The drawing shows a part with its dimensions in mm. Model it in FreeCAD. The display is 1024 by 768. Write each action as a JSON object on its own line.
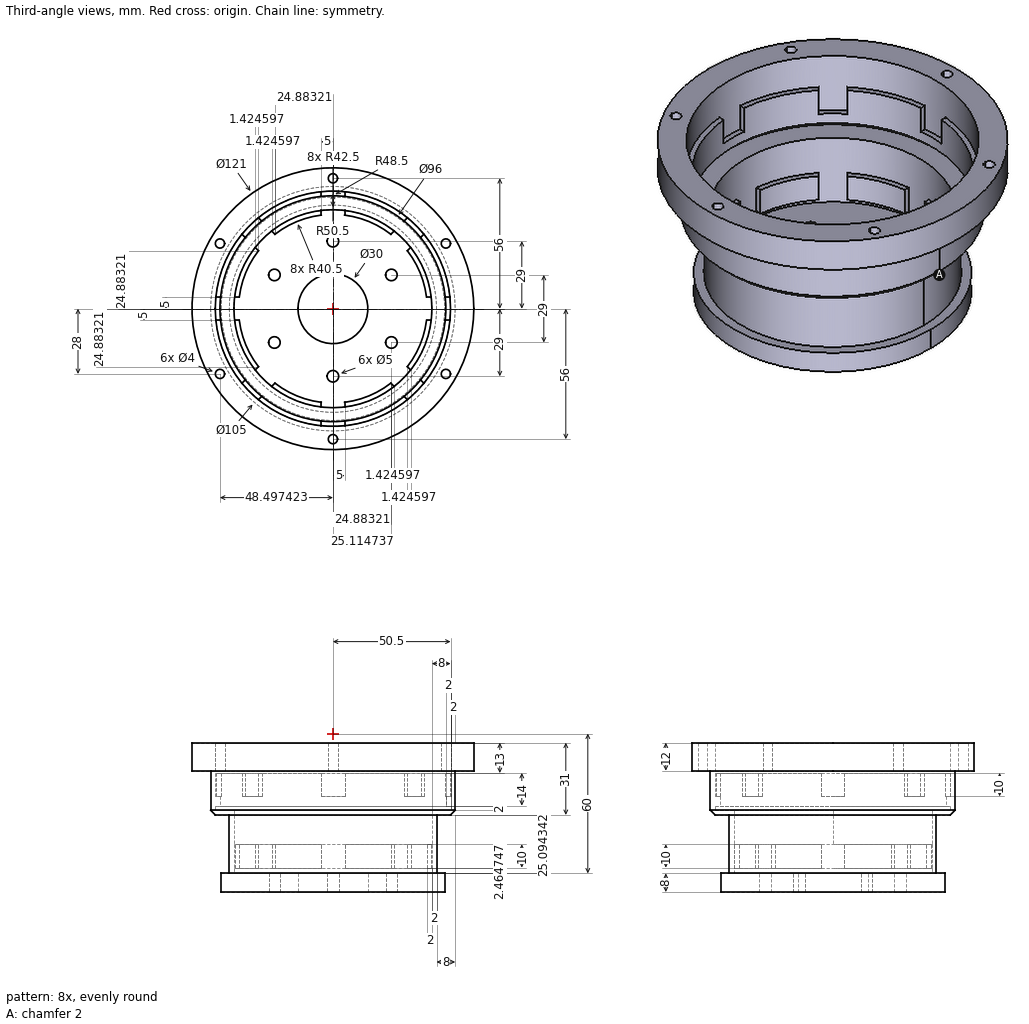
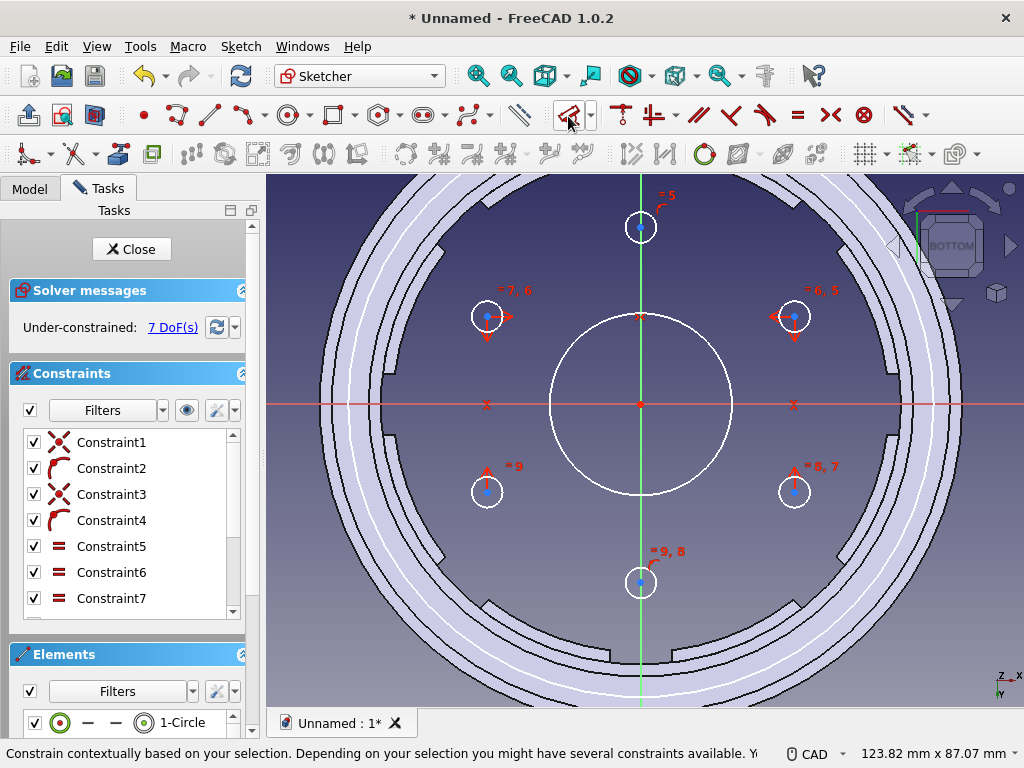
{"action": "left_click", "coordinate": [435, 612]}
{"action": "left_click", "coordinate": [412, 635]}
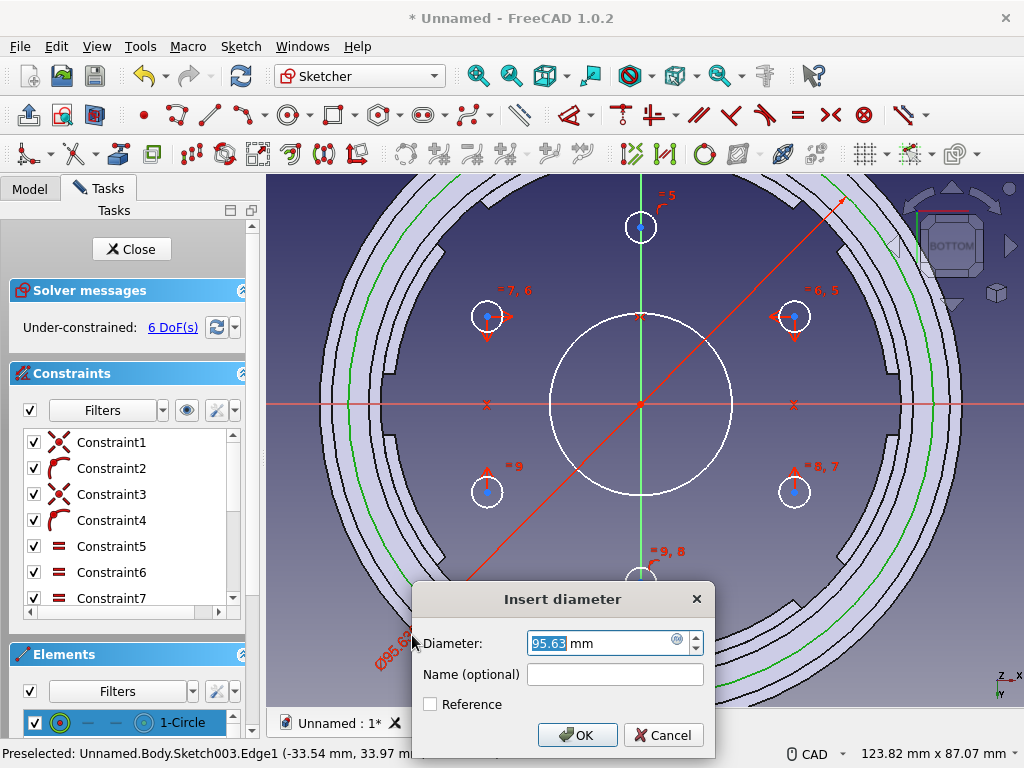
{"action": "type", "text": "96"}
{"action": "key", "text": "Return"}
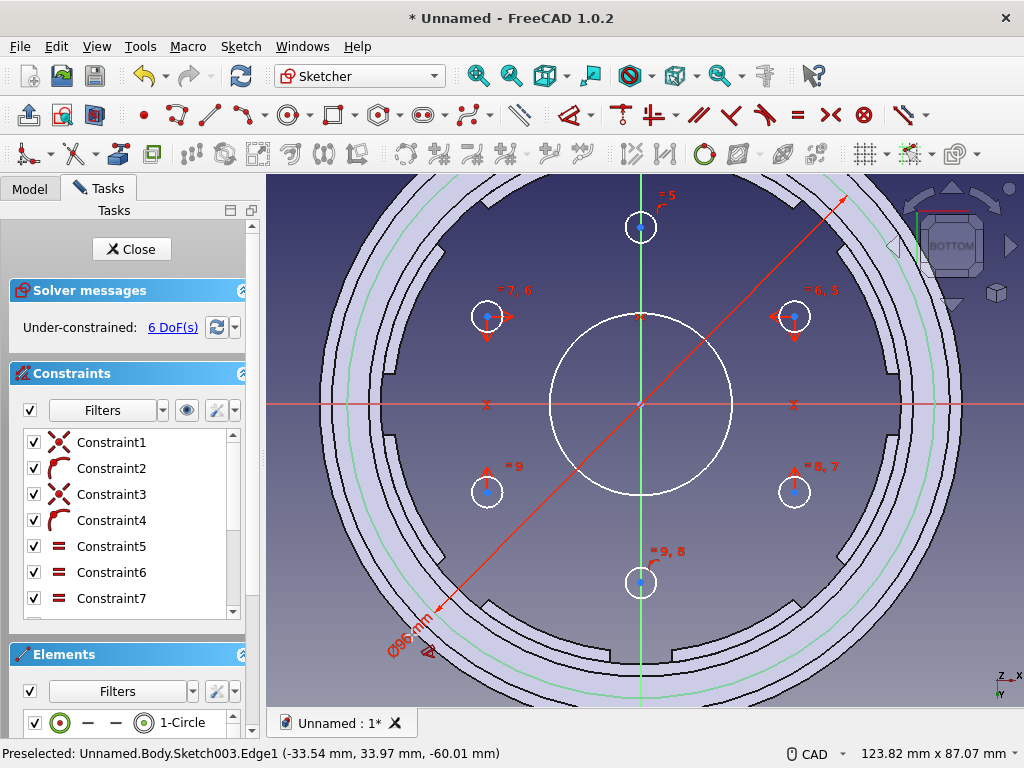
{"action": "scroll", "coordinate": [652, 217], "scroll_direction": "up", "scroll_amount": 2}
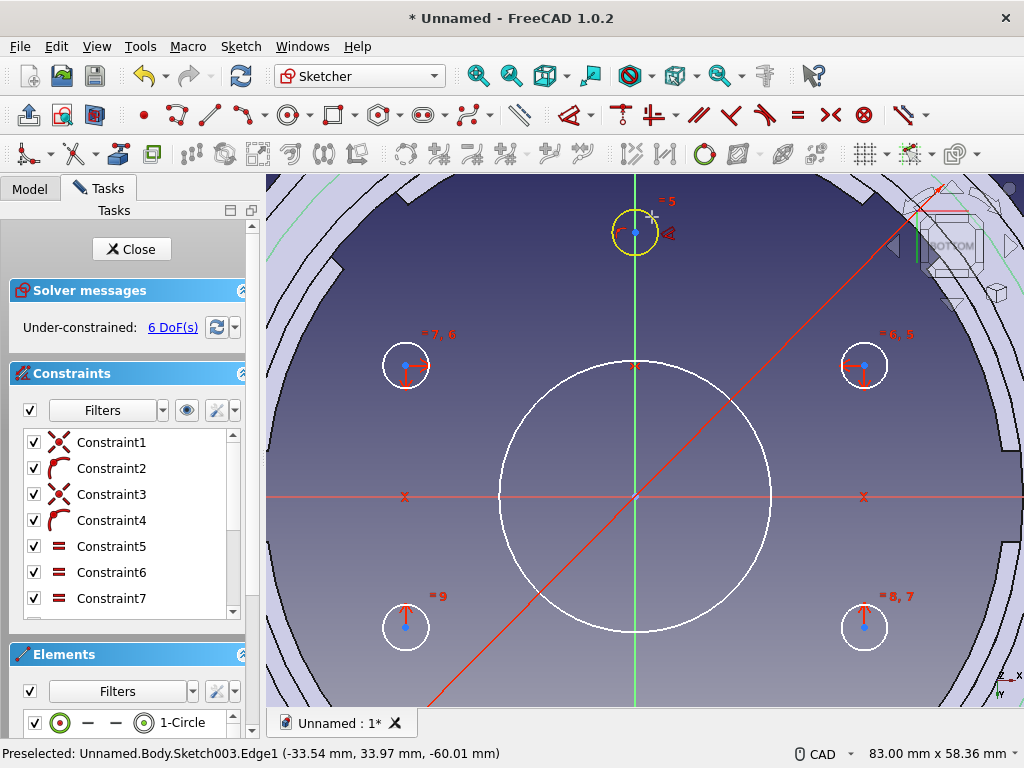
{"action": "left_click", "coordinate": [651, 216]}
{"action": "left_click", "coordinate": [687, 216]}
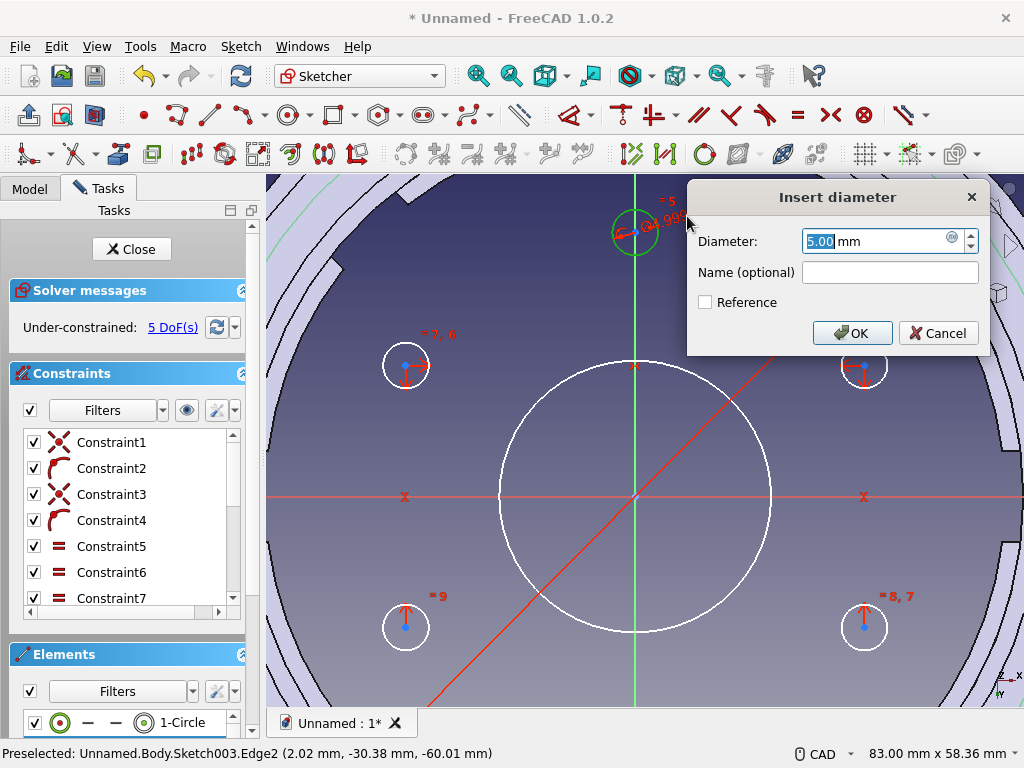
{"action": "type", "text": "5"}
{"action": "key", "text": "Return"}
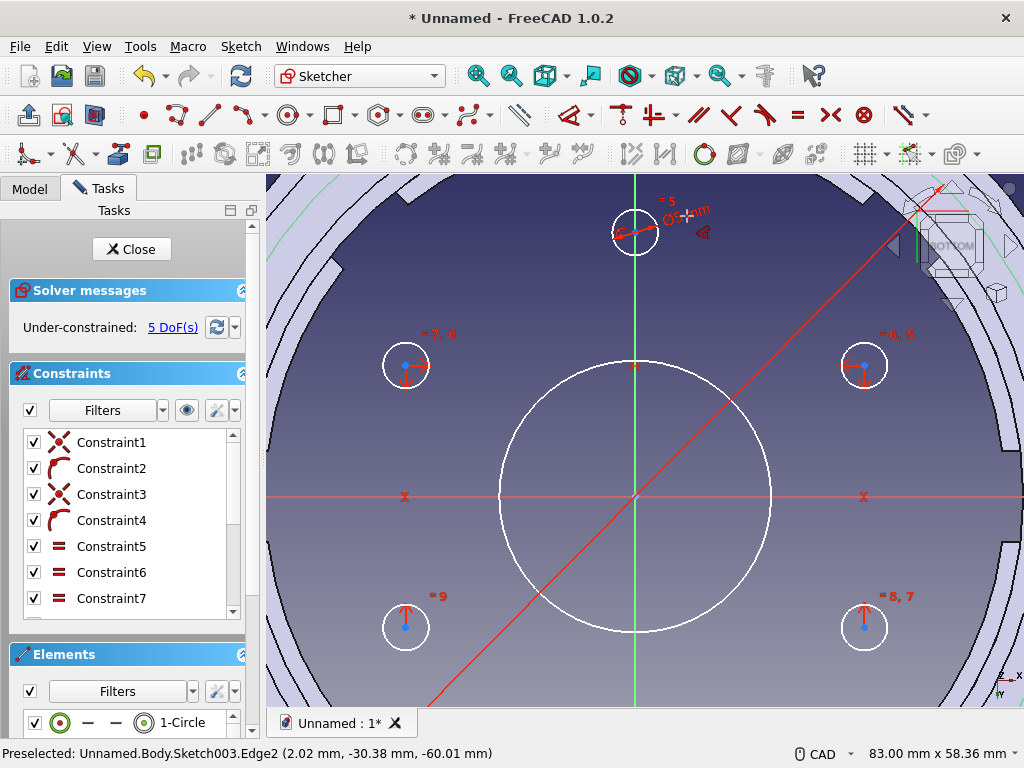
{"action": "left_click", "coordinate": [731, 400]}
{"action": "left_click", "coordinate": [754, 377]}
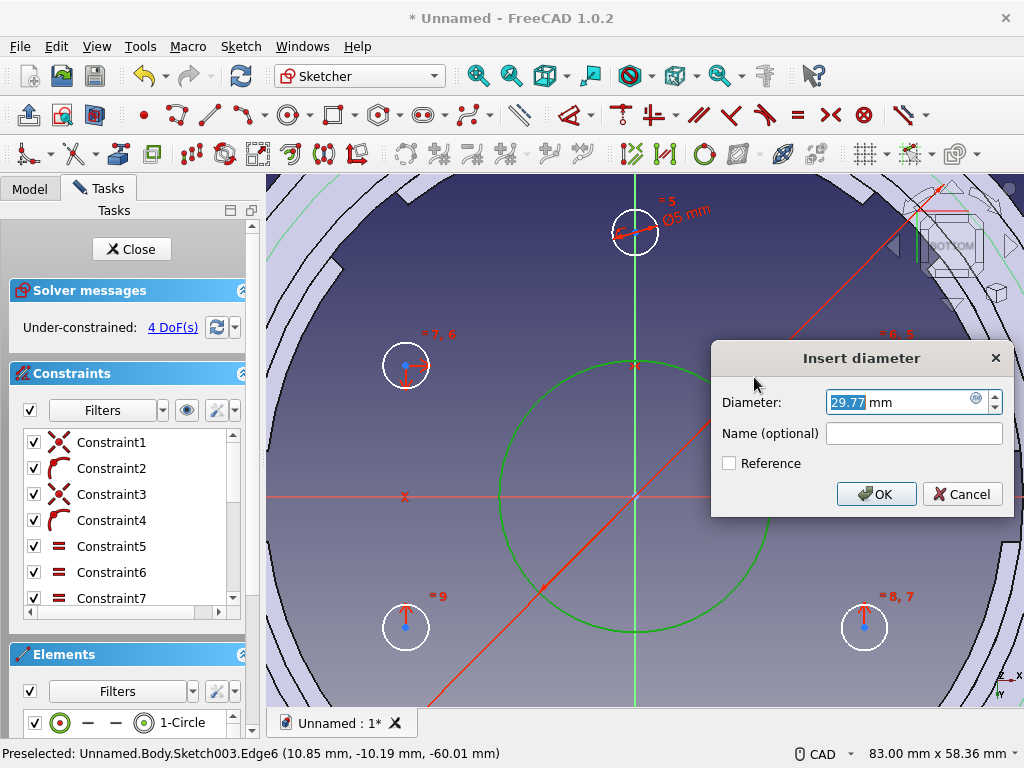
{"action": "type", "text": "30"}
{"action": "key", "text": "Return"}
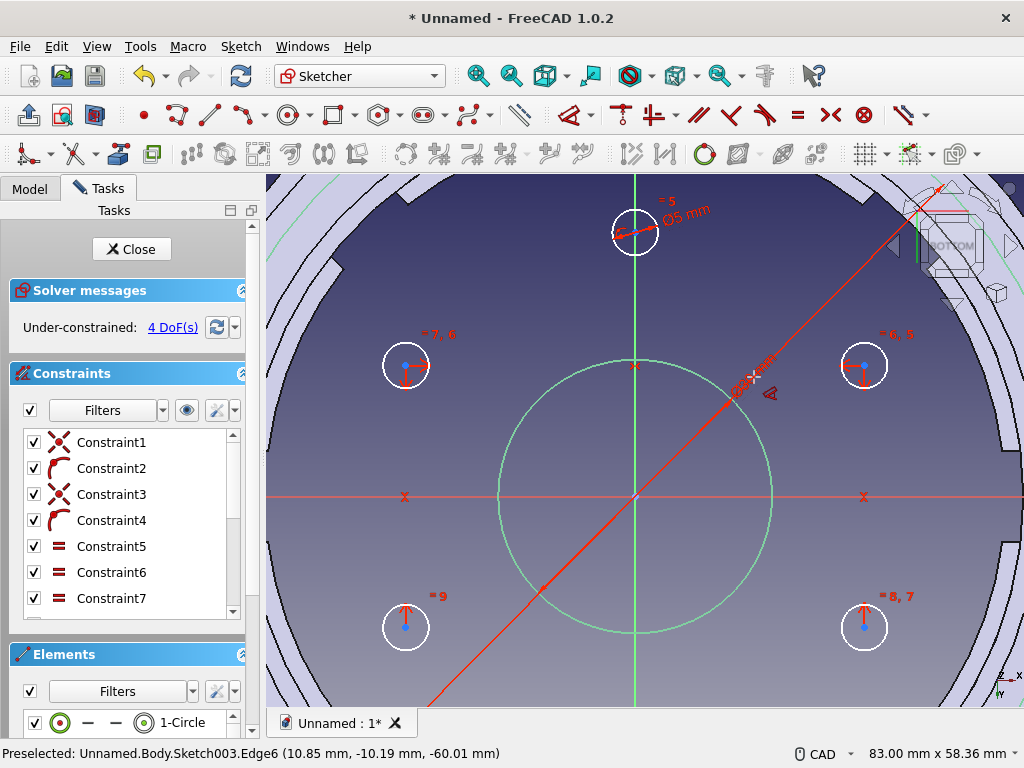
{"action": "left_click", "coordinate": [635, 233]}
{"action": "left_click", "coordinate": [669, 304]}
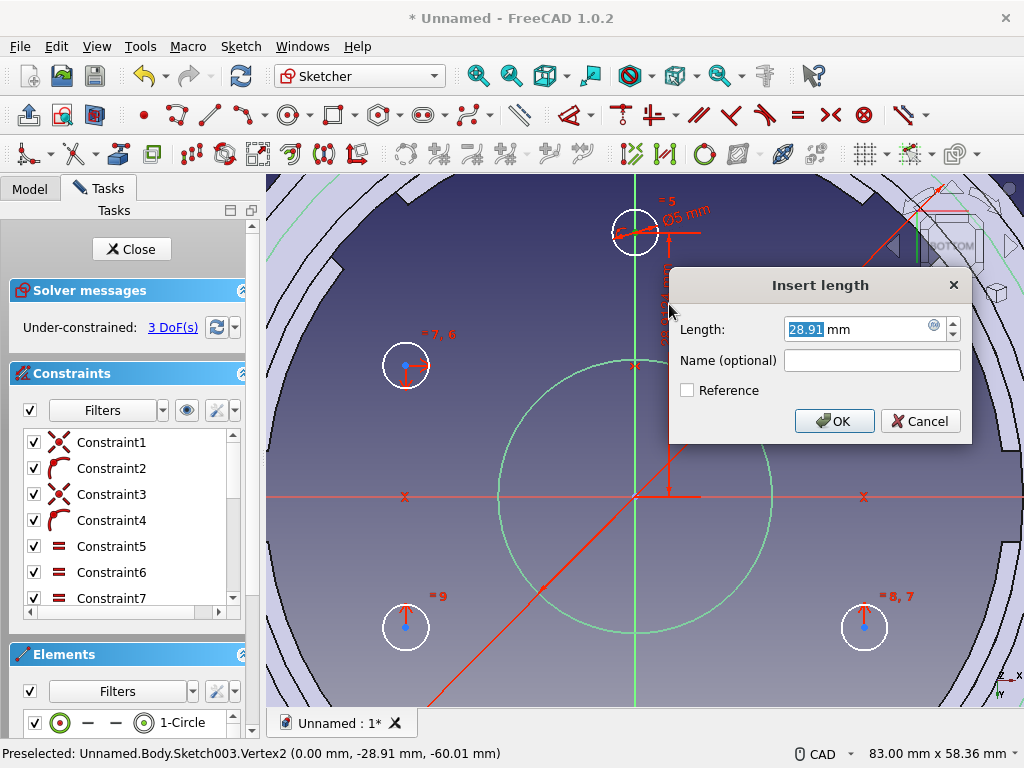
{"action": "type", "text": "29"}
{"action": "key", "text": "Return"}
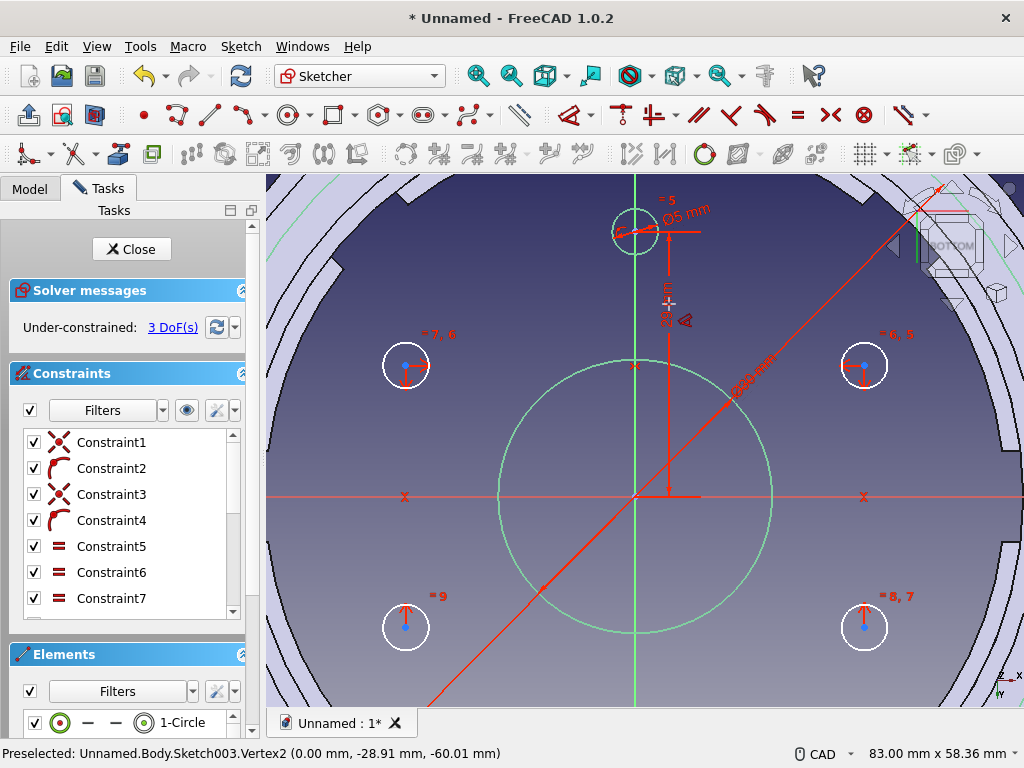
{"action": "scroll", "coordinate": [542, 408], "scroll_direction": "down", "scroll_amount": 5}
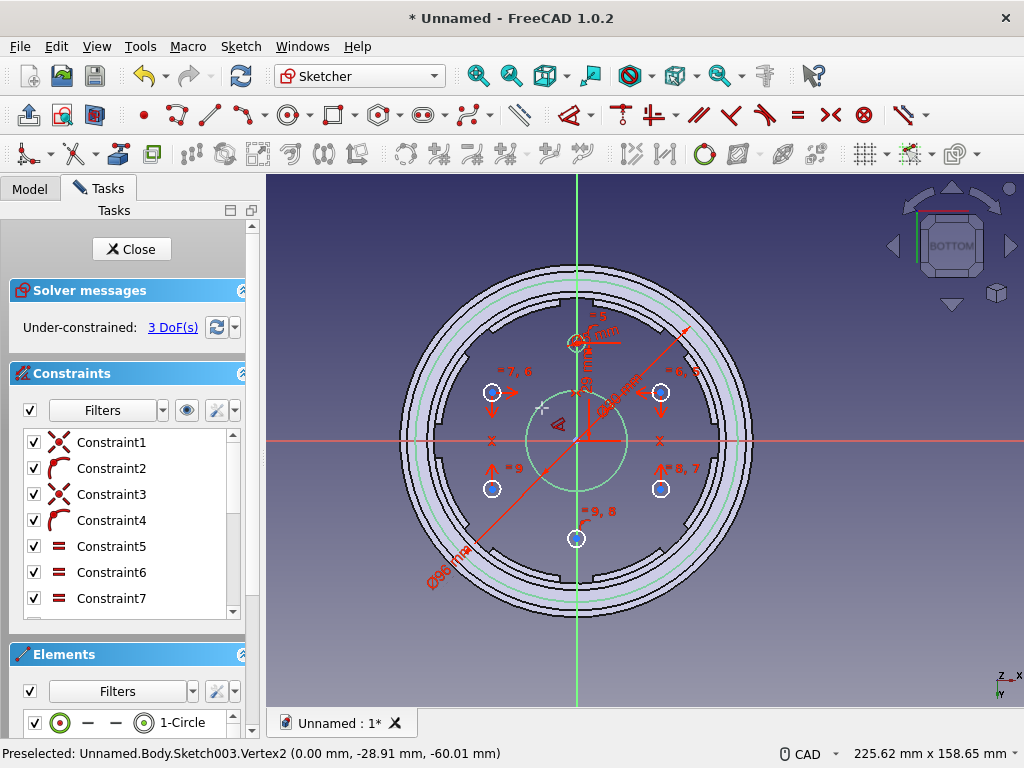
{"action": "left_click", "coordinate": [577, 539]}
{"action": "left_click", "coordinate": [611, 512]}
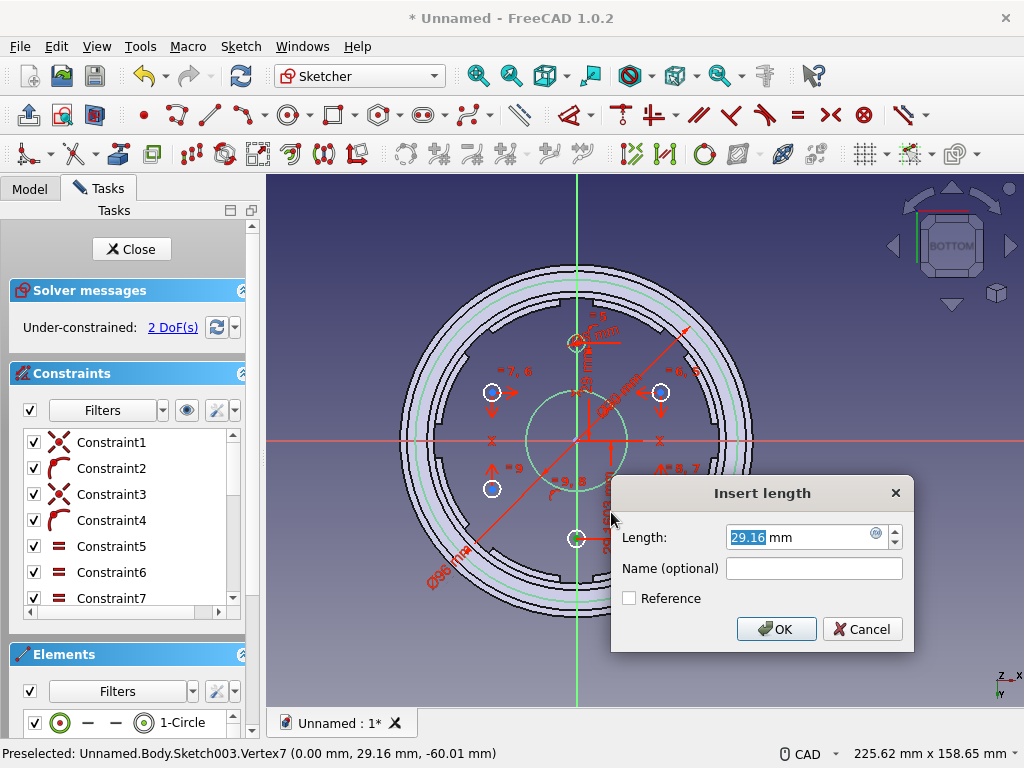
{"action": "type", "text": "29"}
{"action": "key", "text": "Return"}